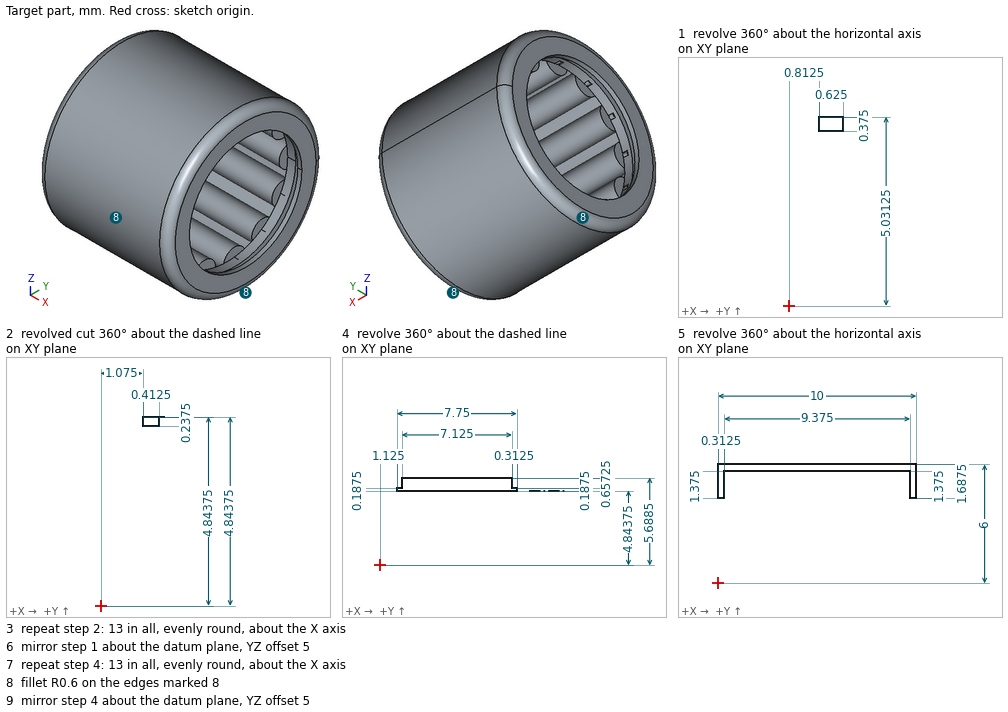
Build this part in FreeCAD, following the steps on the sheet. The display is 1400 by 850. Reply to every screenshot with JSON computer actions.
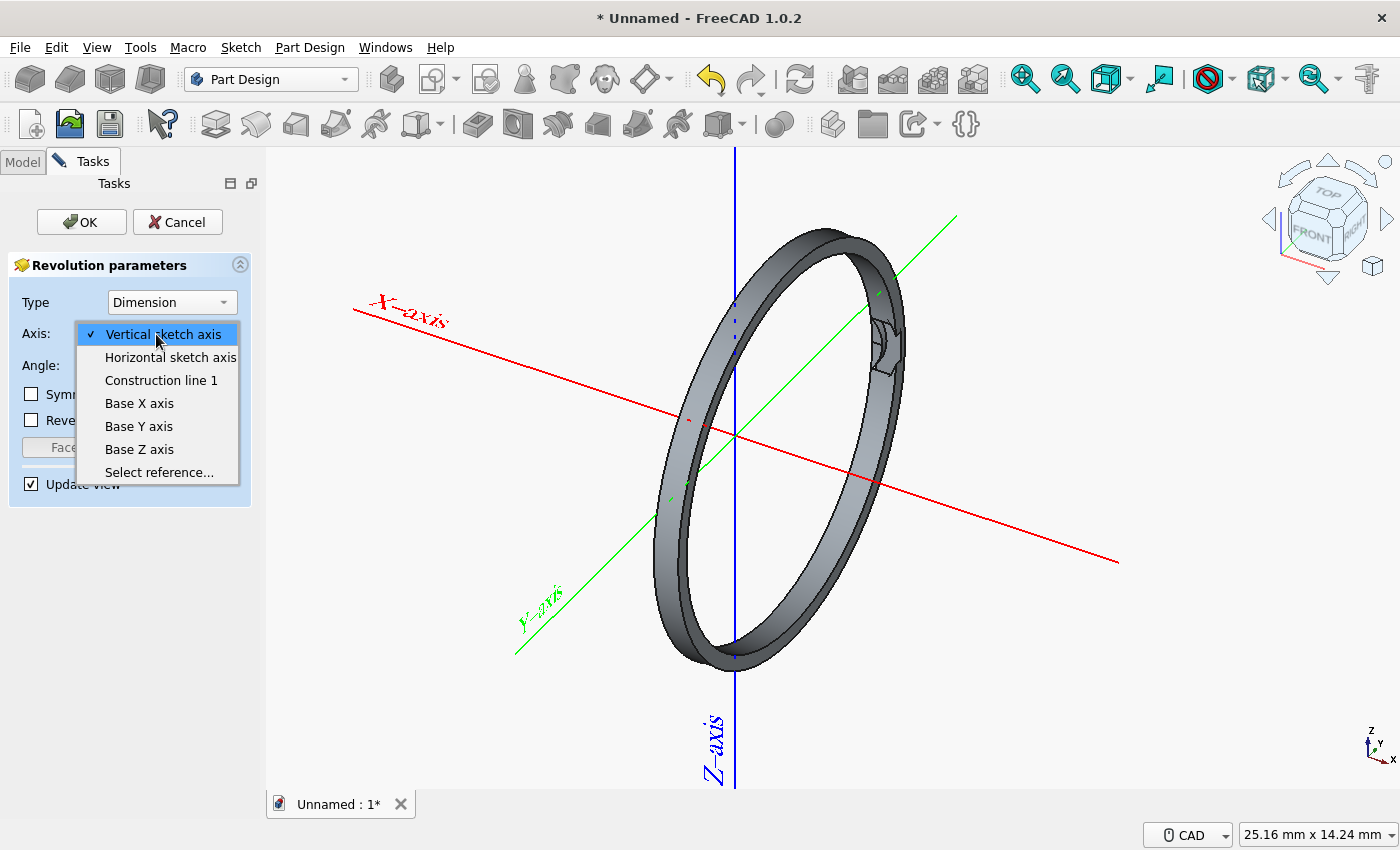
{"action": "left_click", "coordinate": [156, 380]}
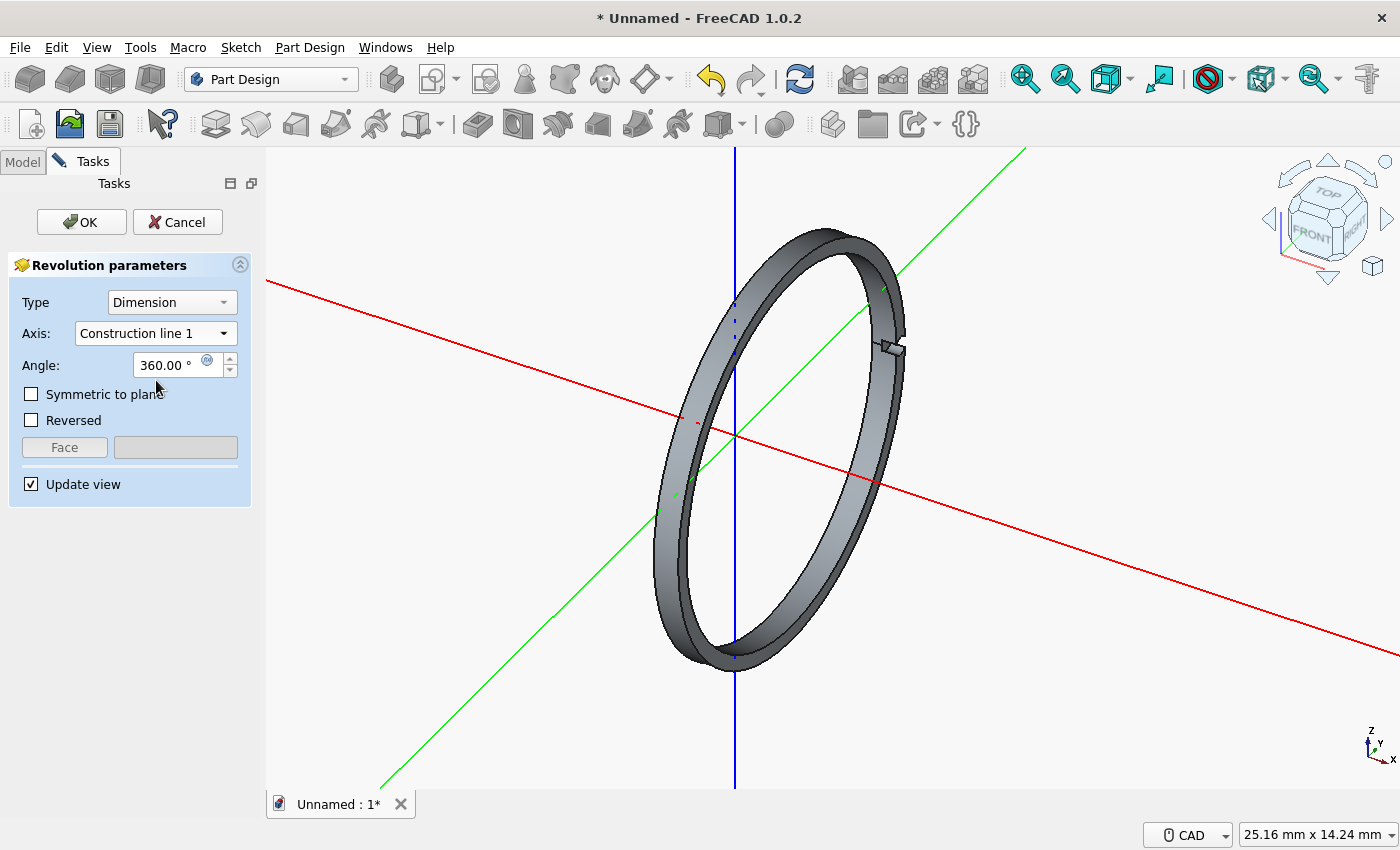
{"action": "left_click", "coordinate": [82, 222]}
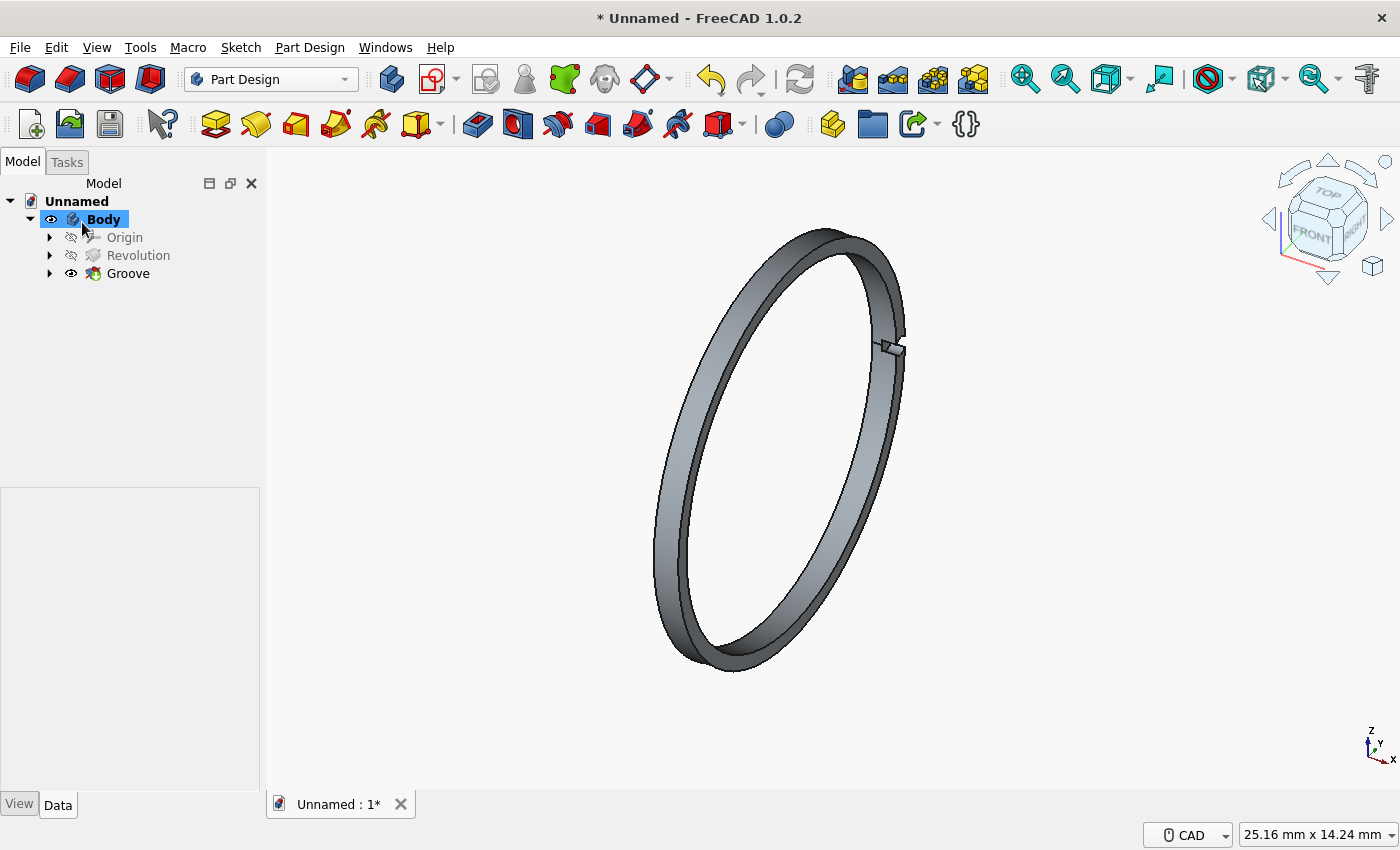
{"action": "left_click", "coordinate": [116, 273]}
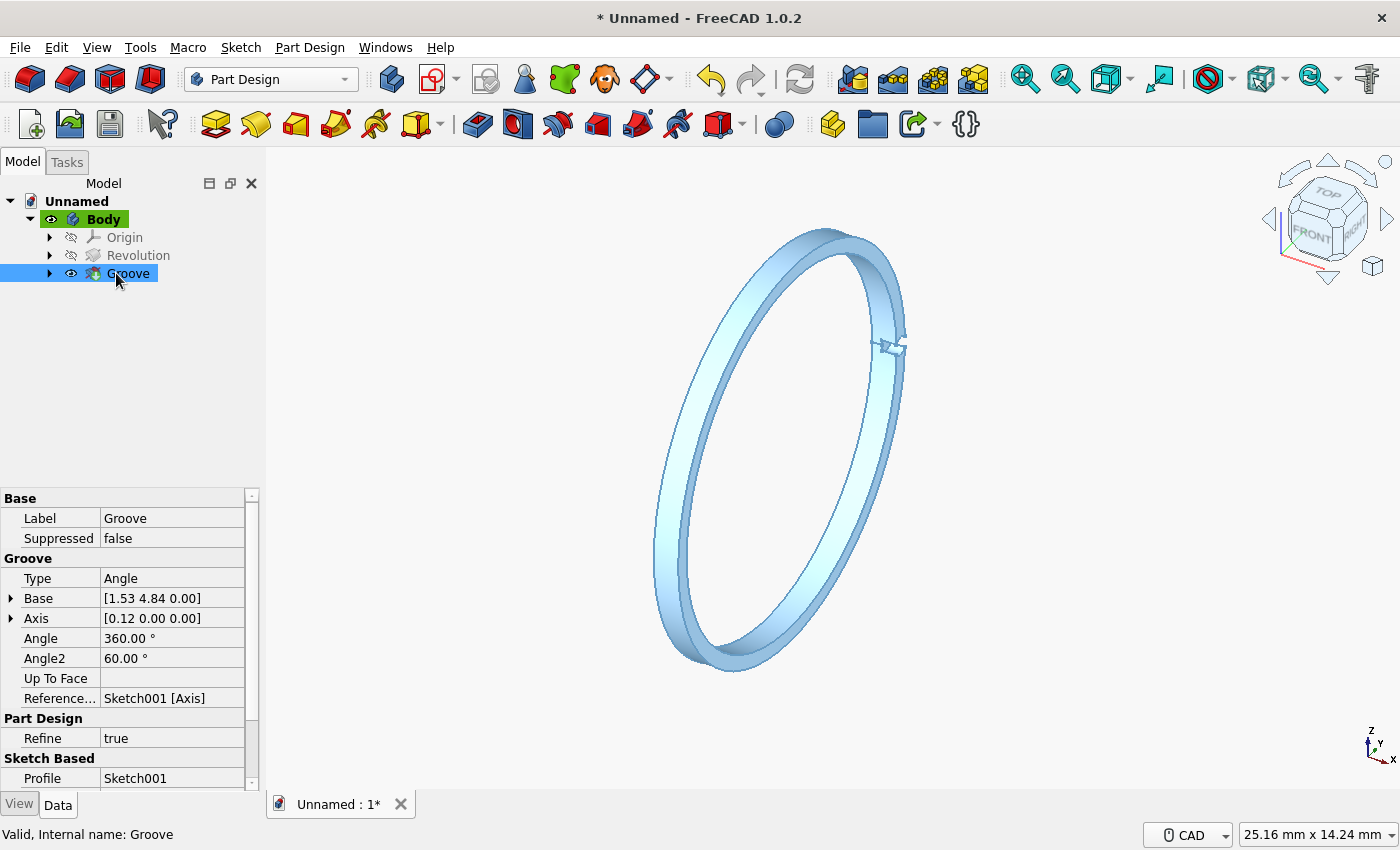
{"action": "left_click", "coordinate": [934, 80]}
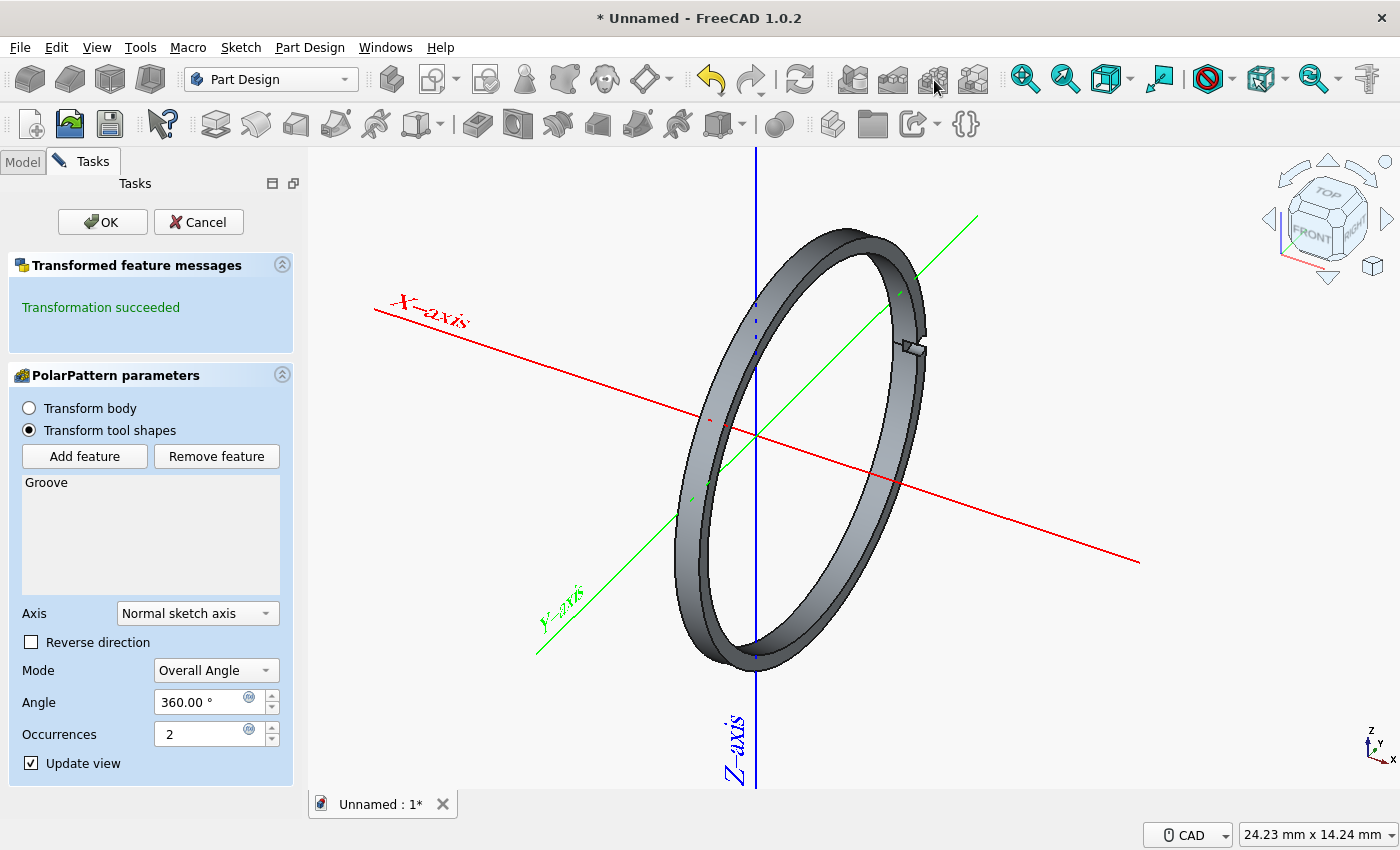
{"action": "left_click", "coordinate": [198, 614]}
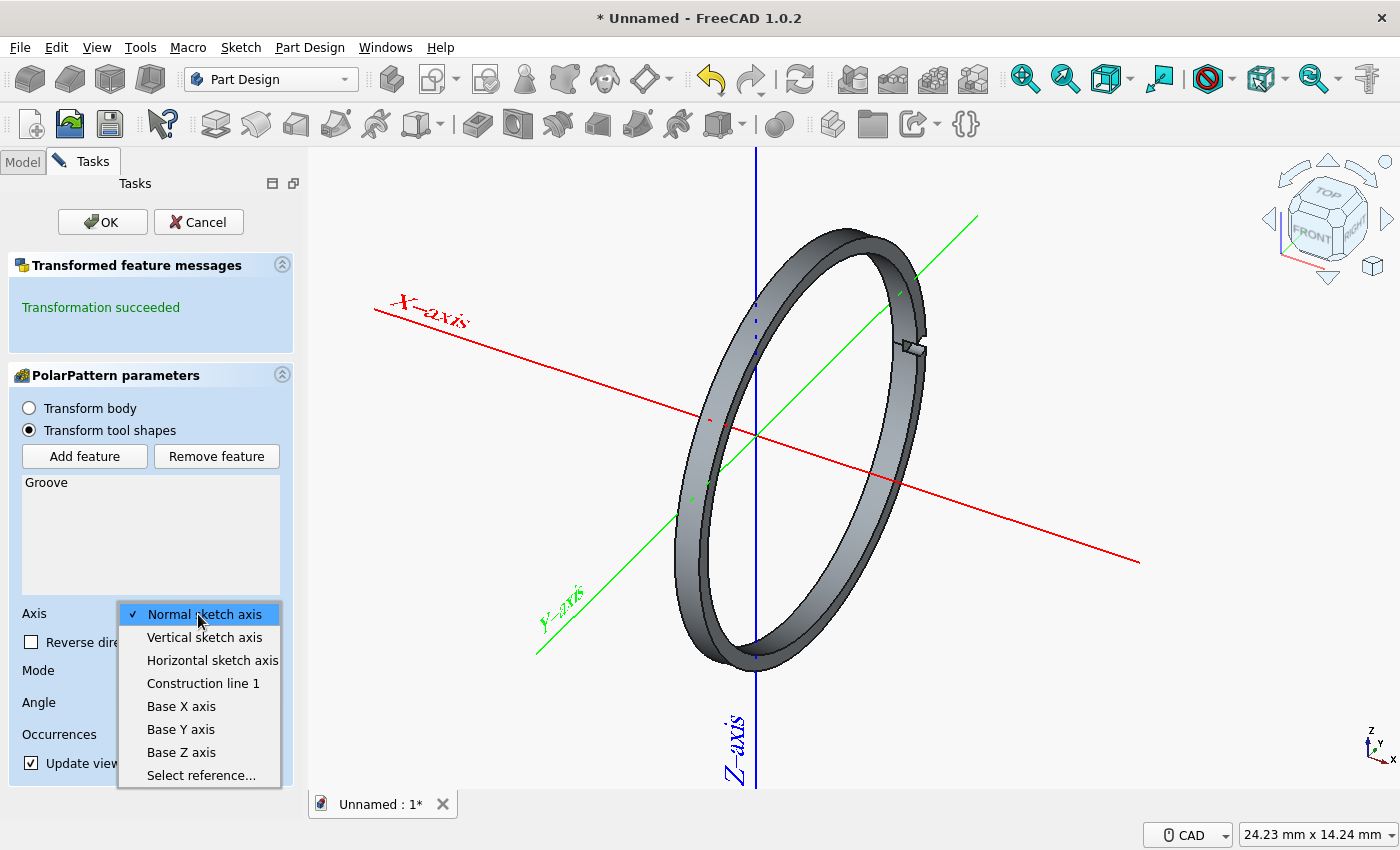
{"action": "left_click", "coordinate": [198, 706]}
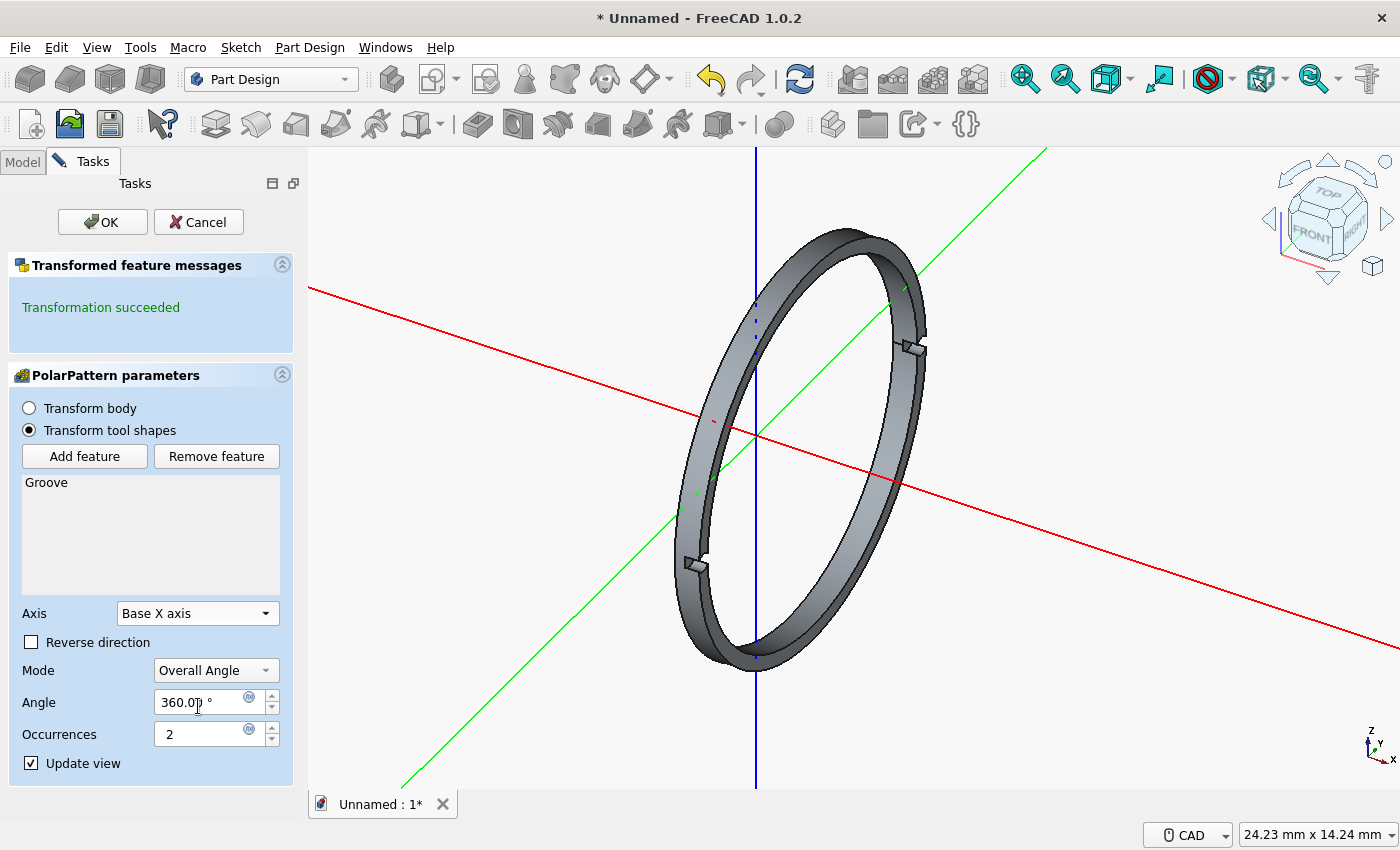
{"action": "triple_click", "coordinate": [209, 734]}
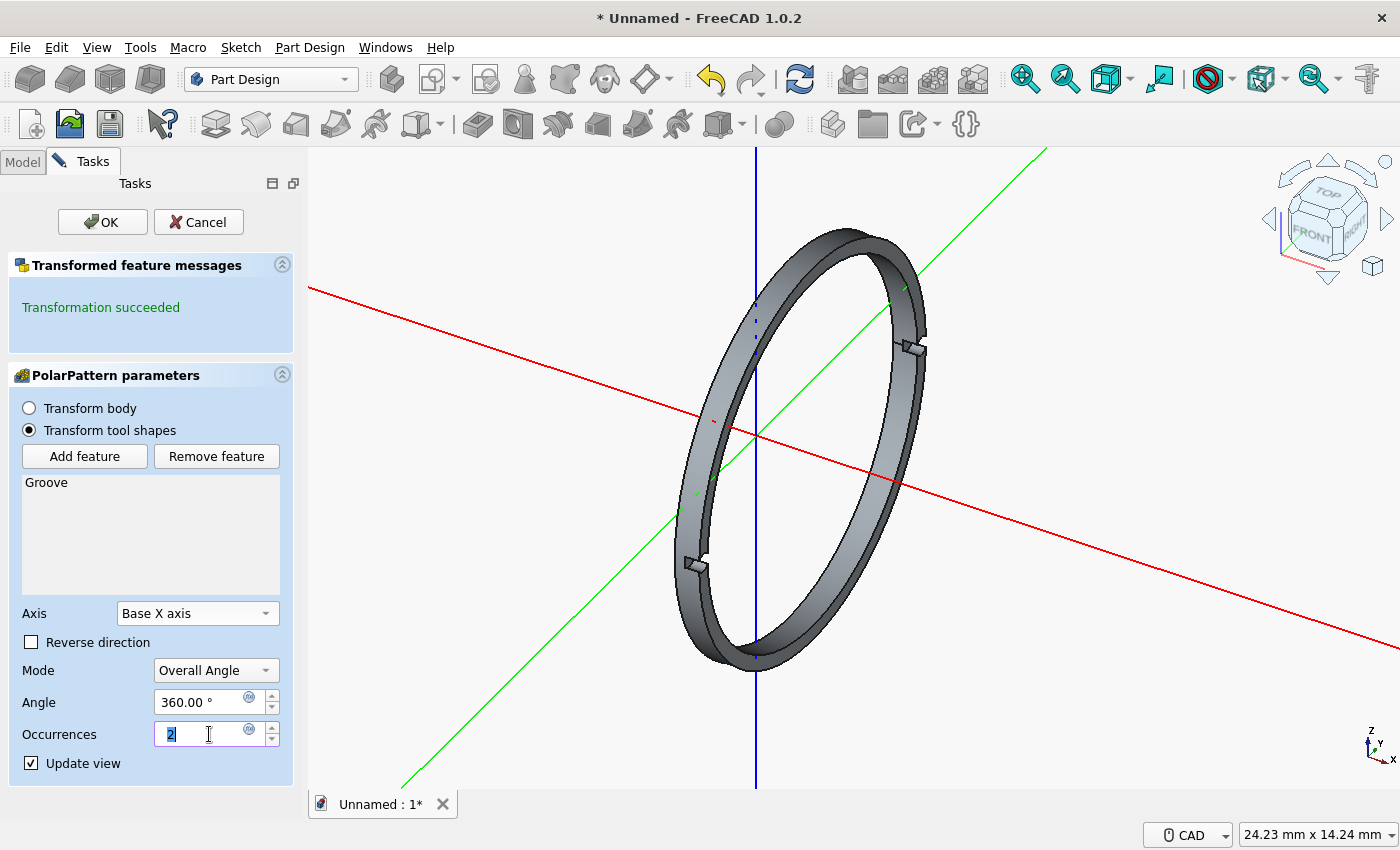
{"action": "type", "text": "13"}
{"action": "key", "text": "Tab"}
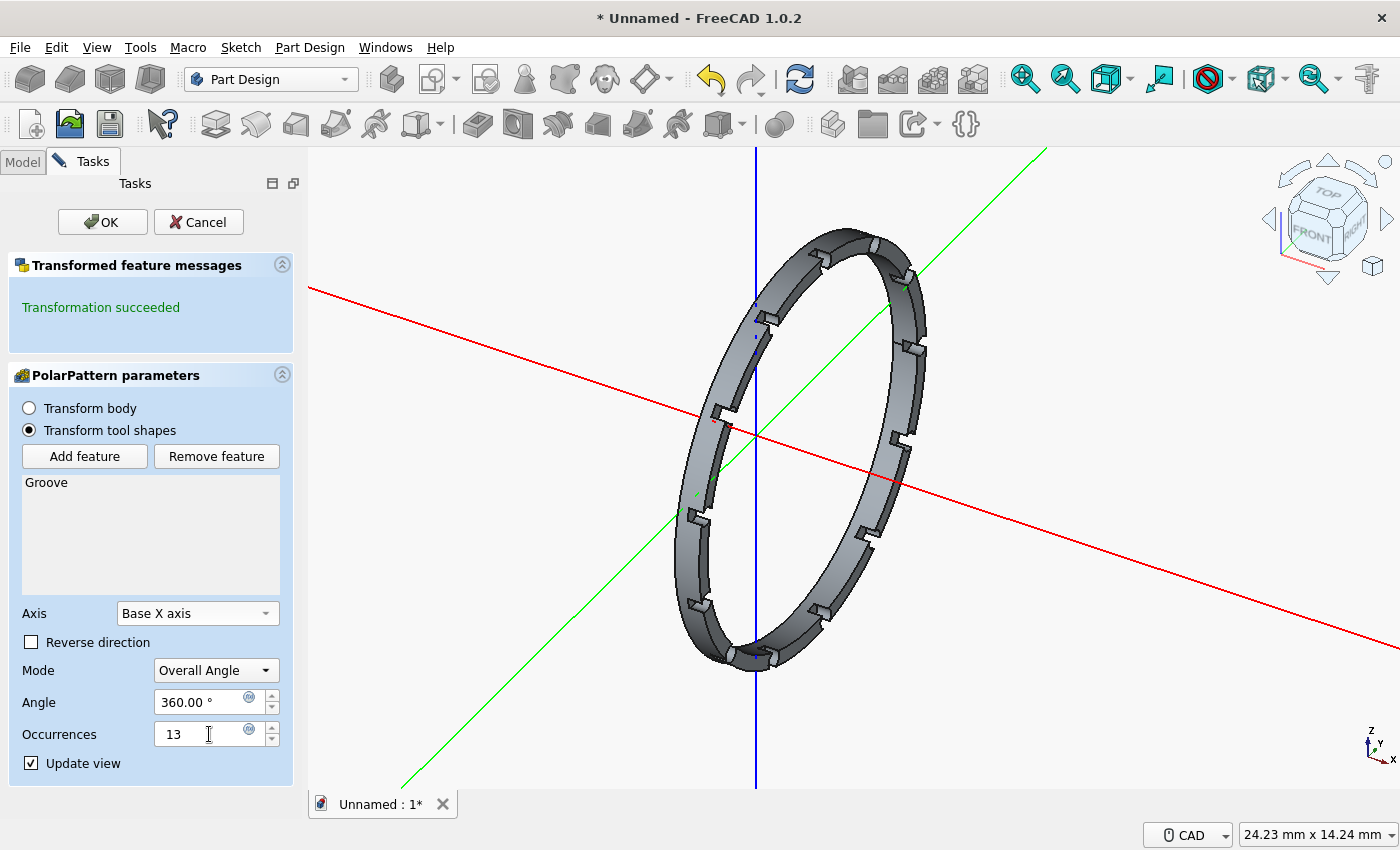
{"action": "left_click", "coordinate": [103, 222]}